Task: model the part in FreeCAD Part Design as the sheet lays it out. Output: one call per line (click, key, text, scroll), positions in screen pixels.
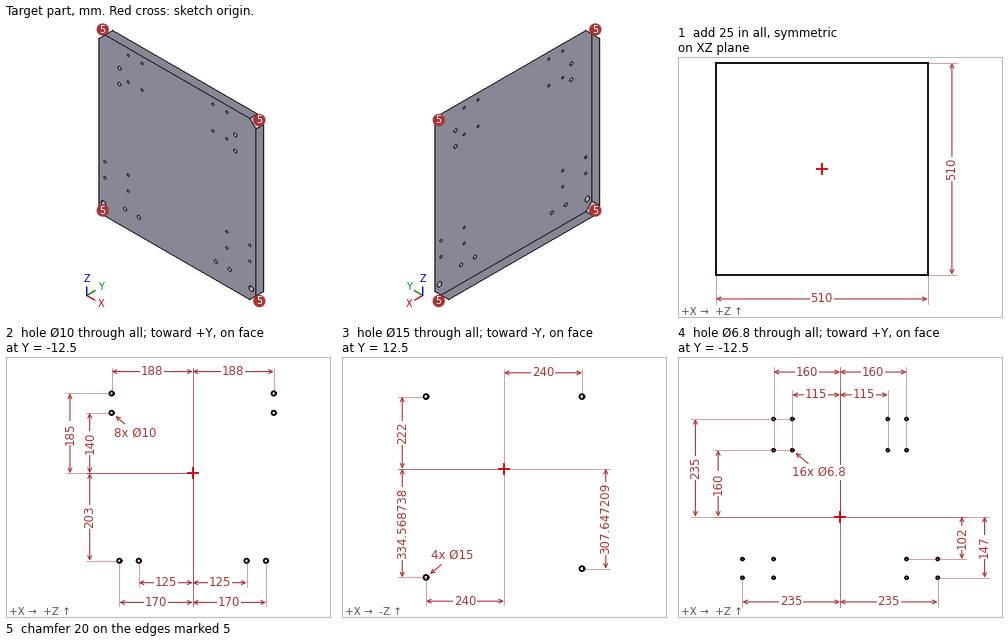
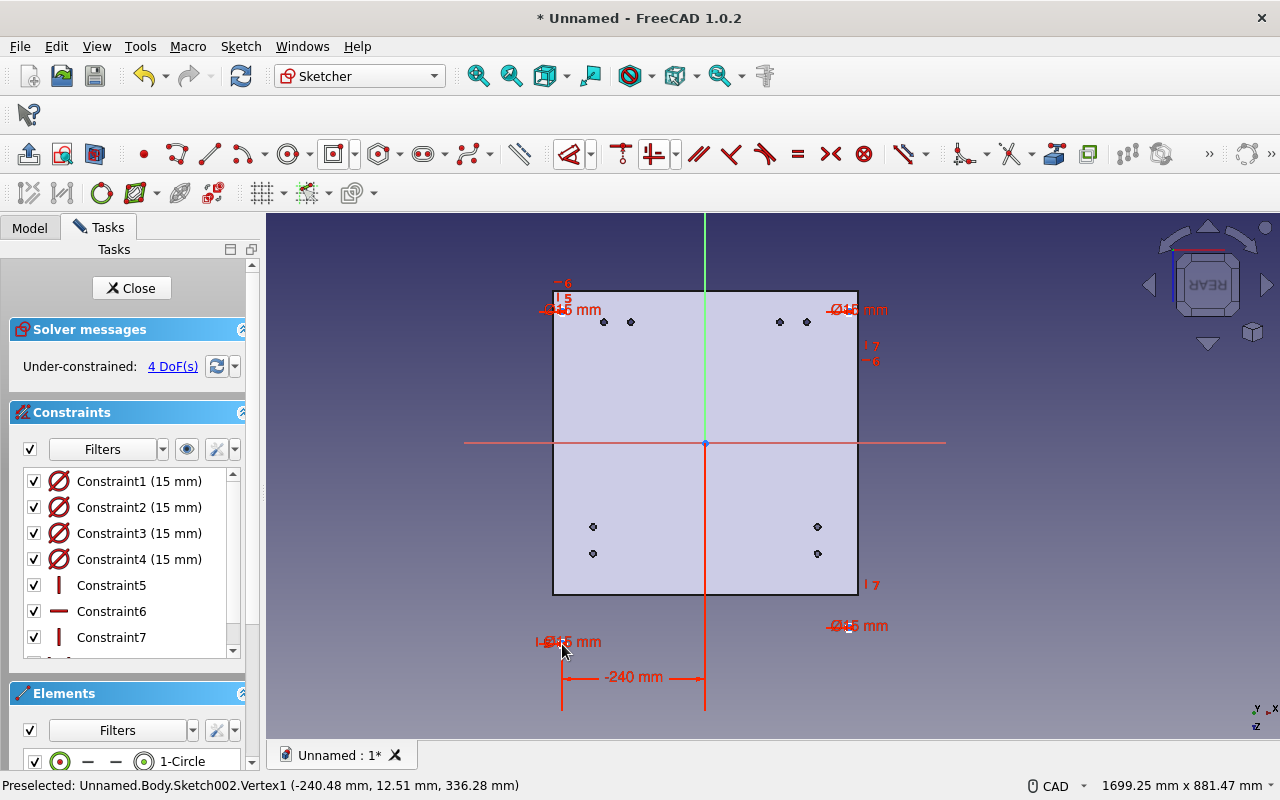
click(562, 312)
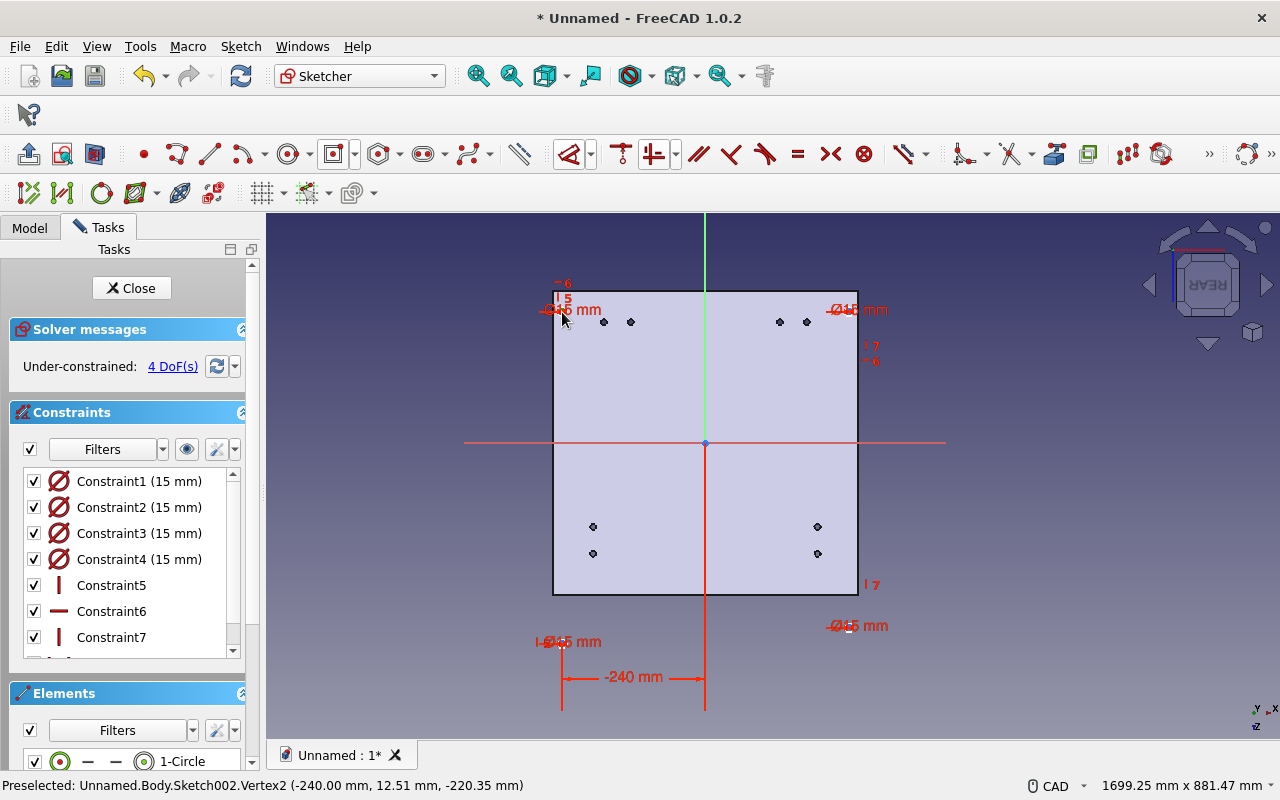
click(590, 154)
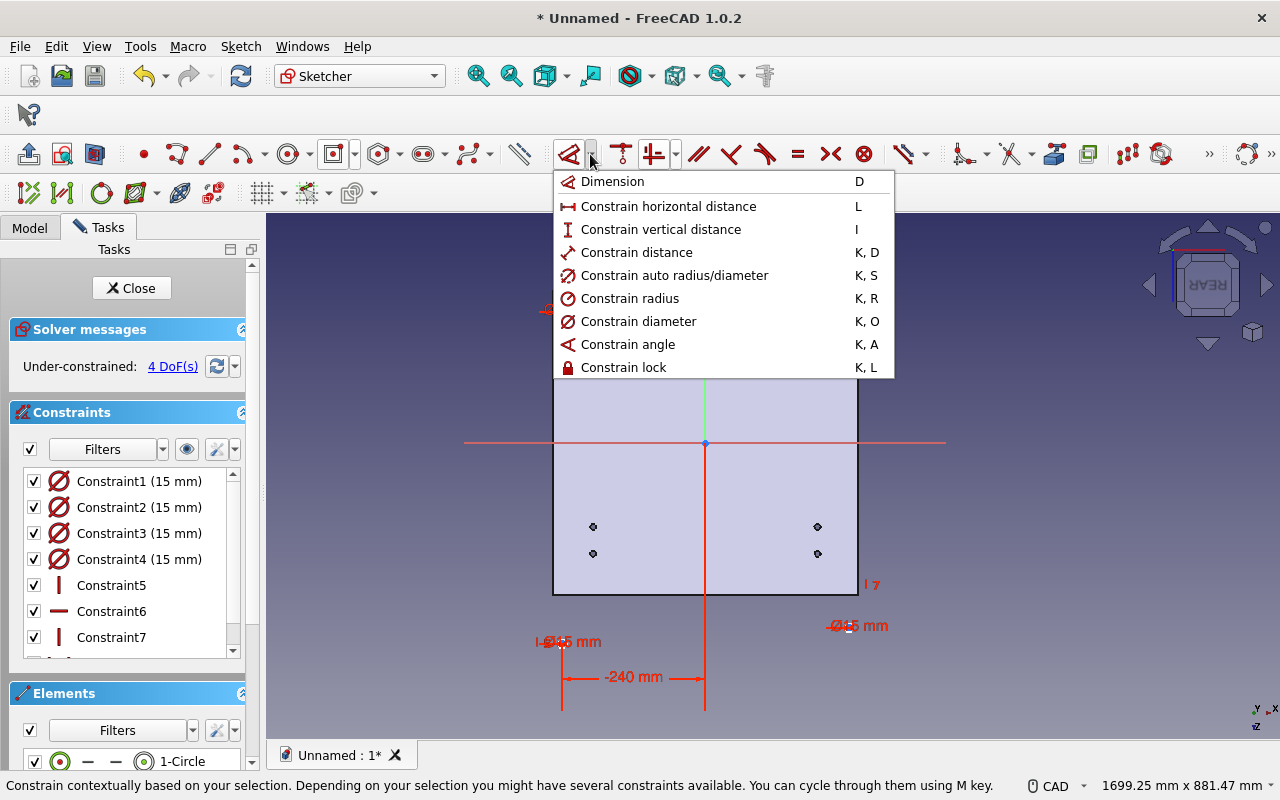
click(724, 230)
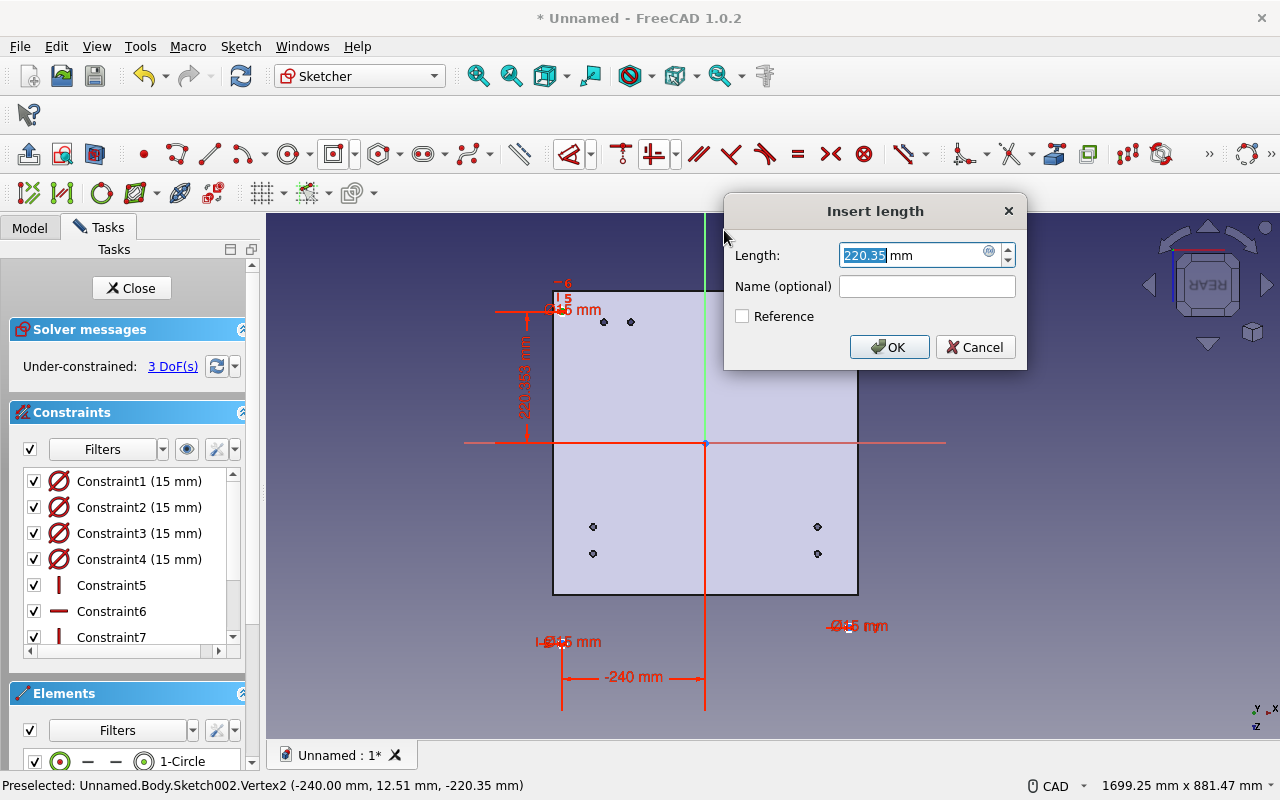
text(222)
key(Return)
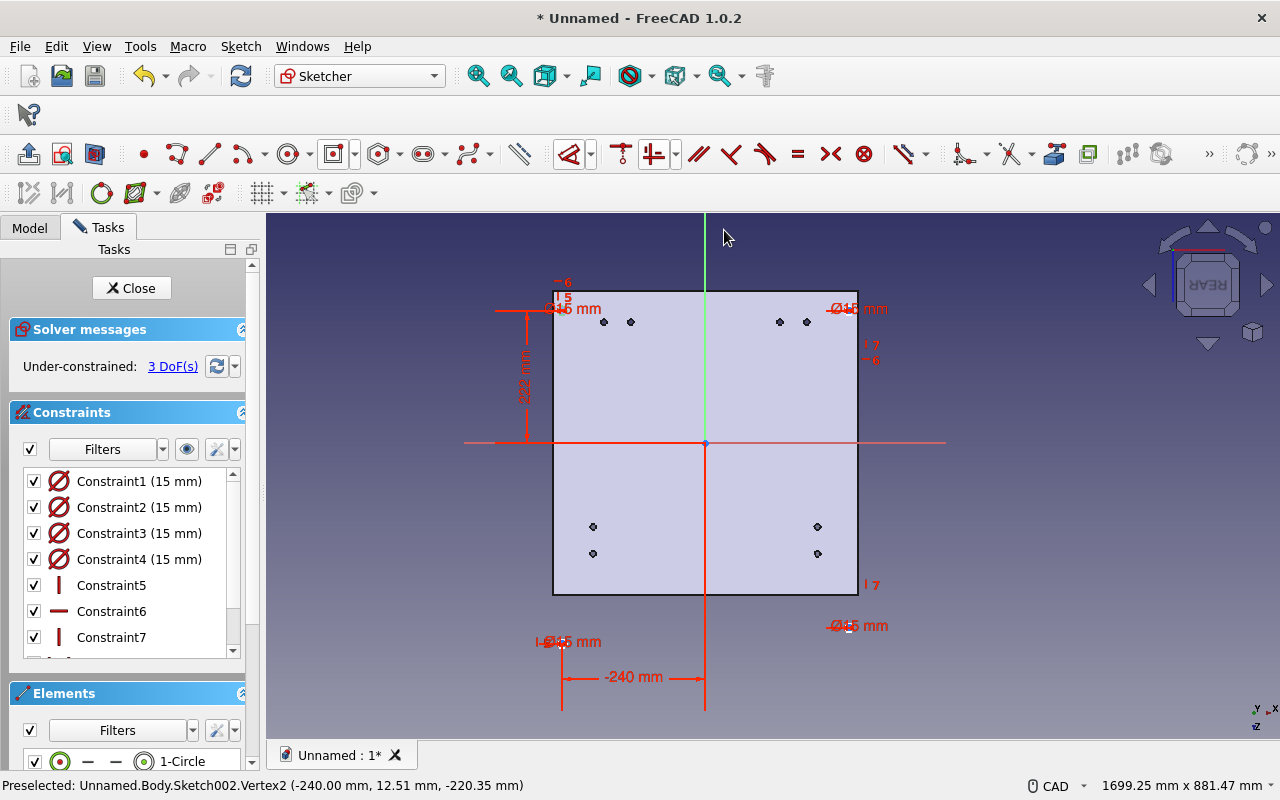
click(849, 311)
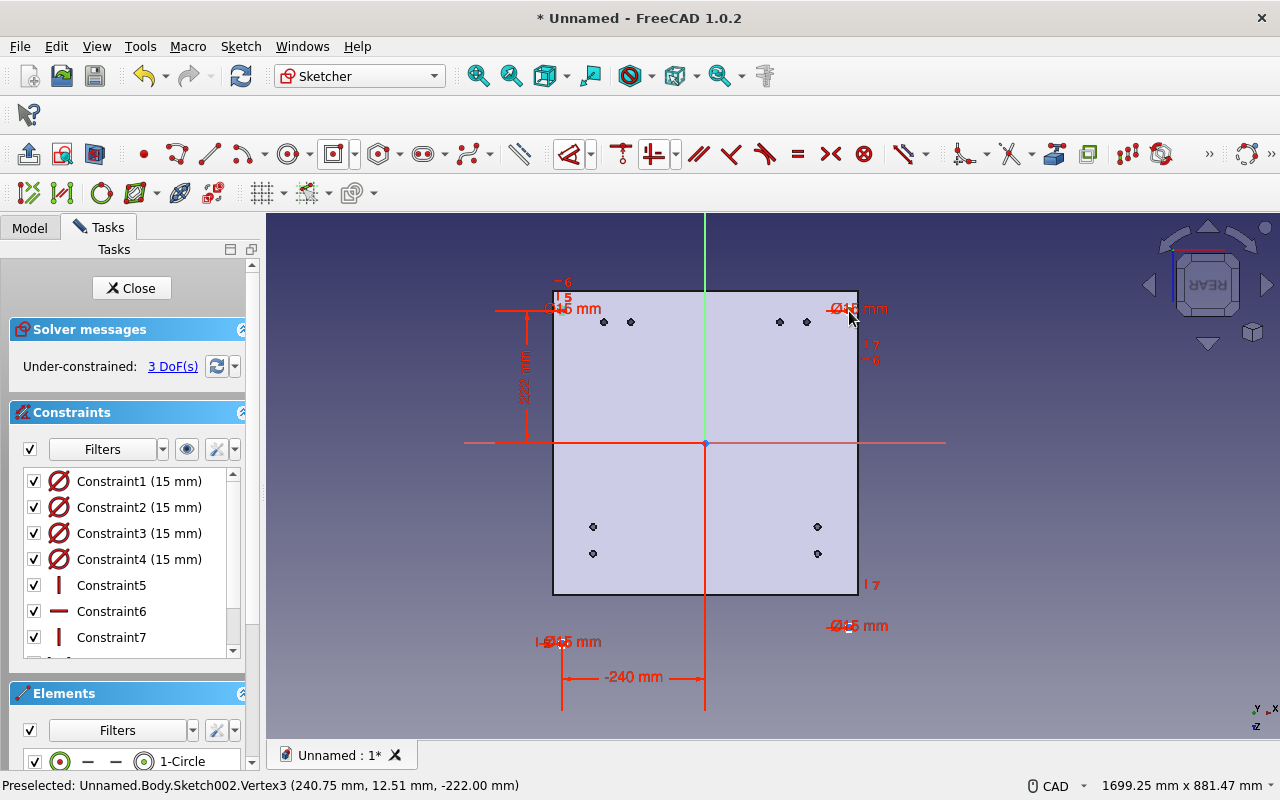
key(l)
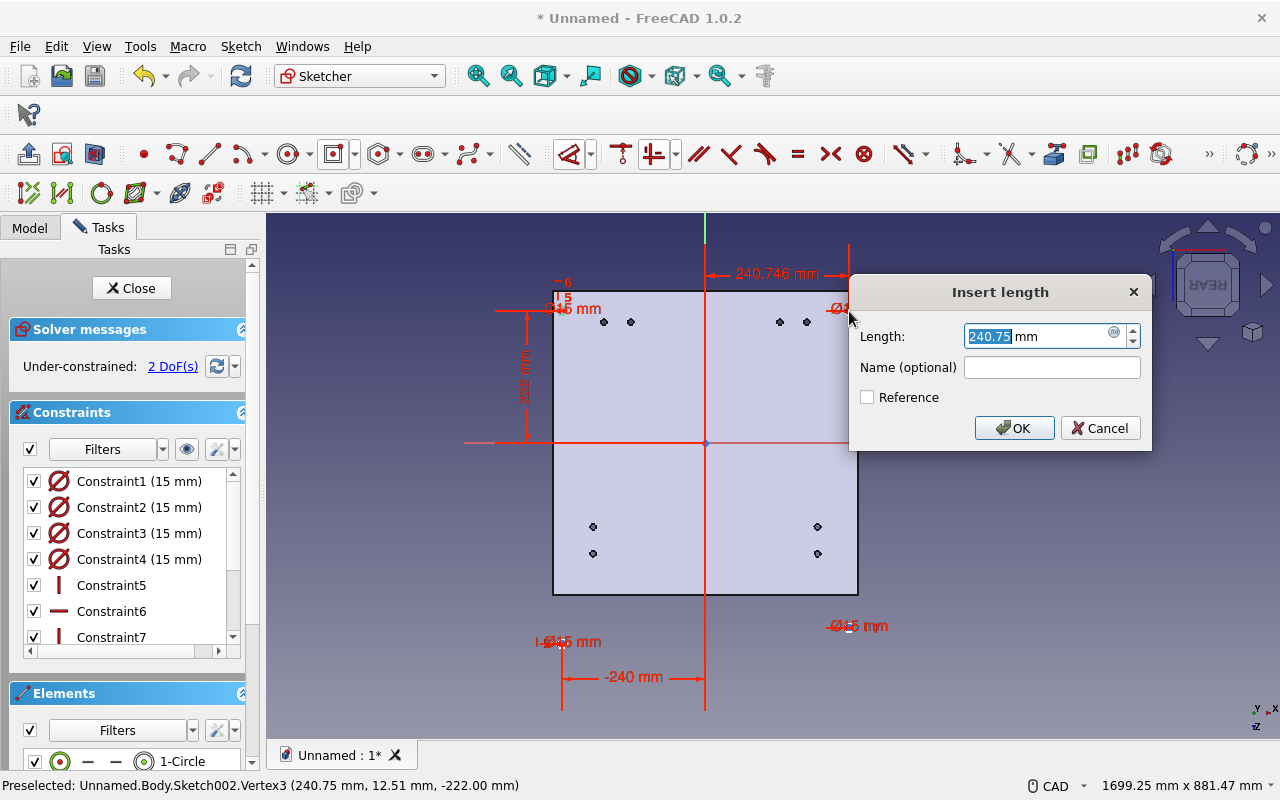
text(240)
key(Return)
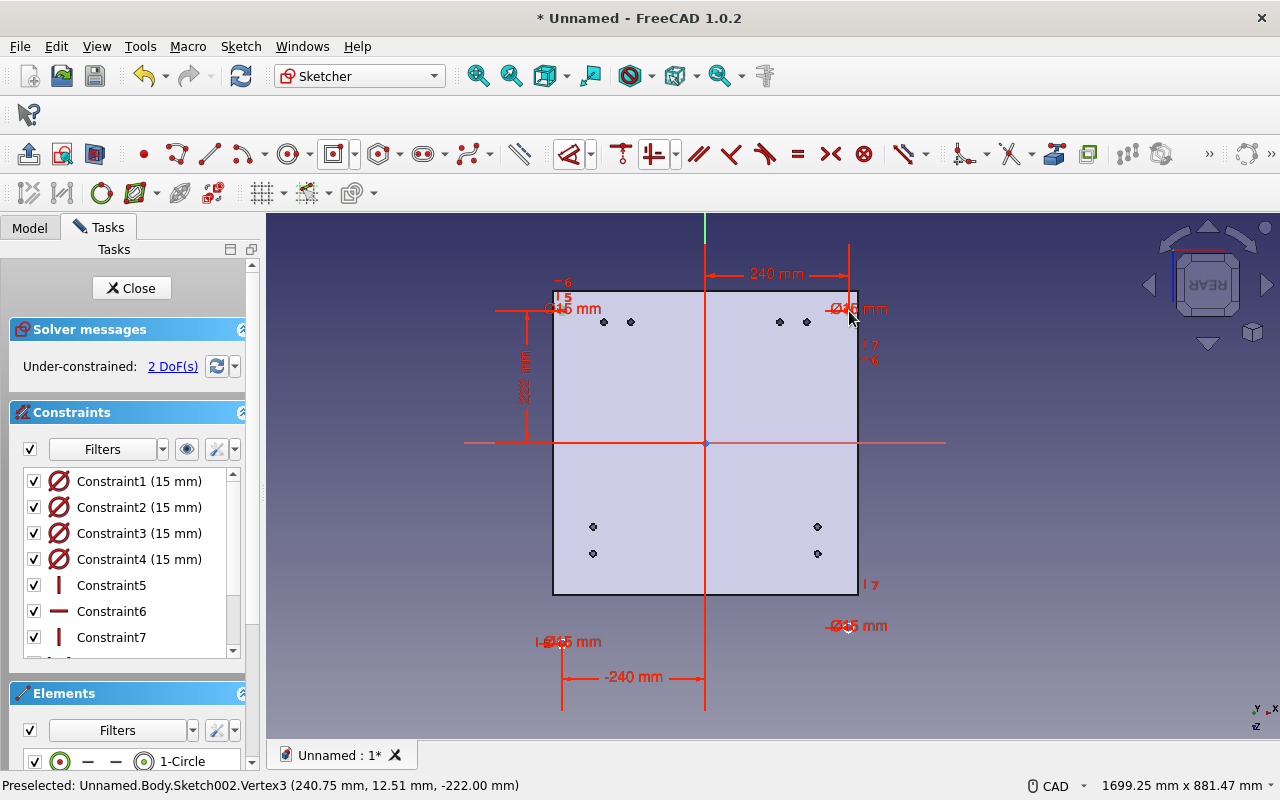
click(562, 644)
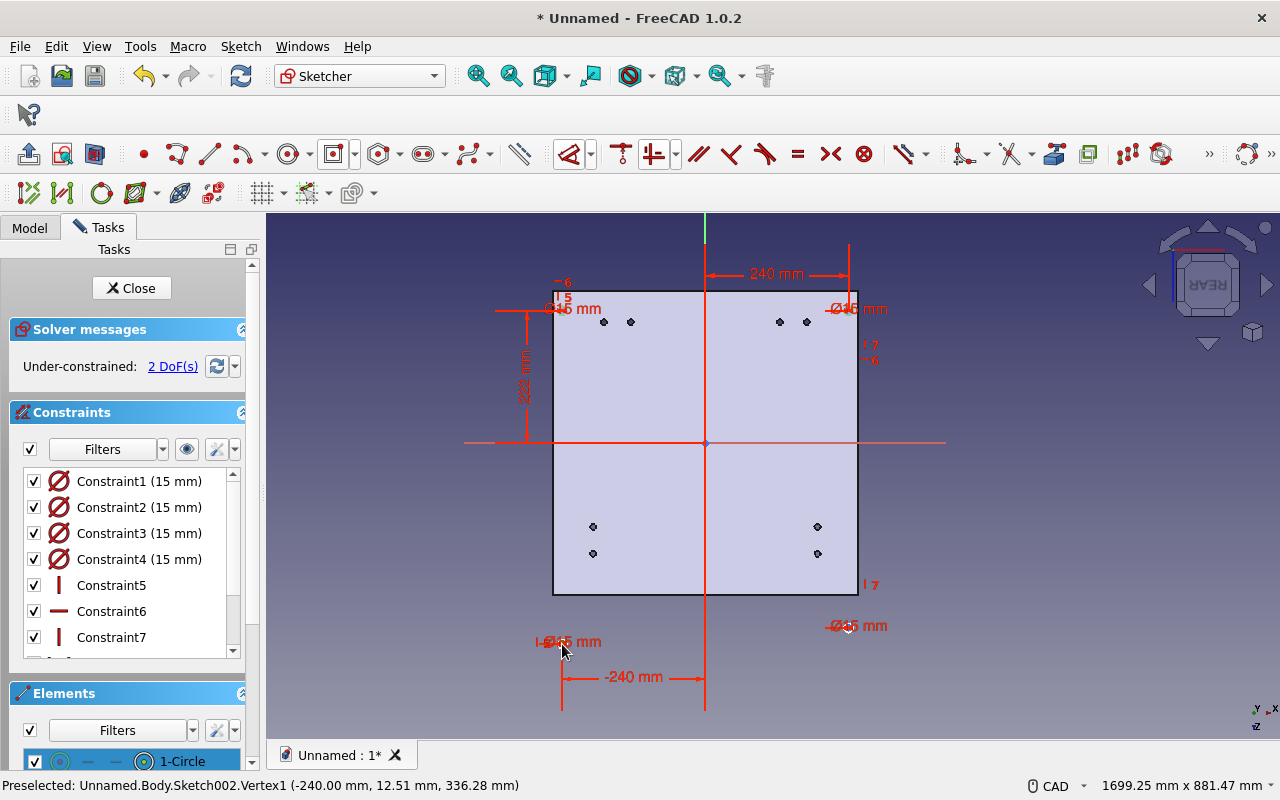
click(590, 154)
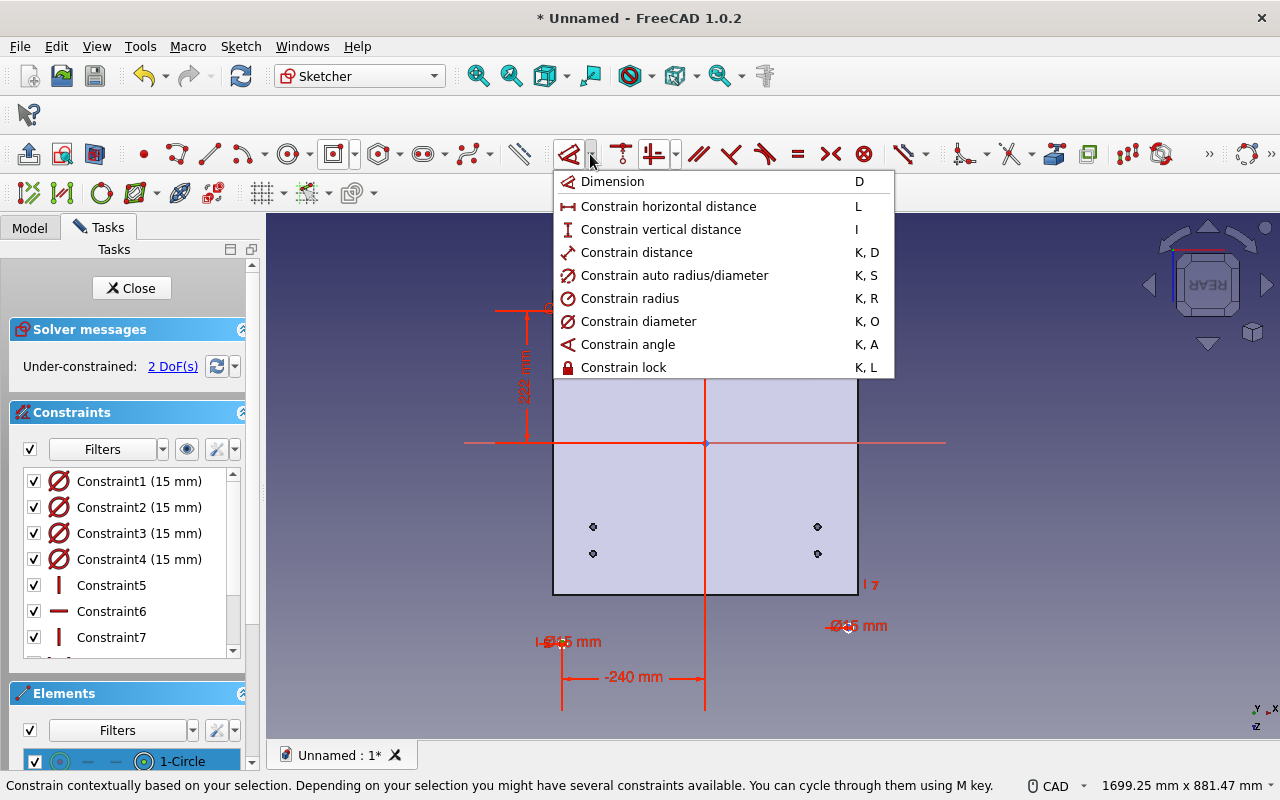
click(724, 230)